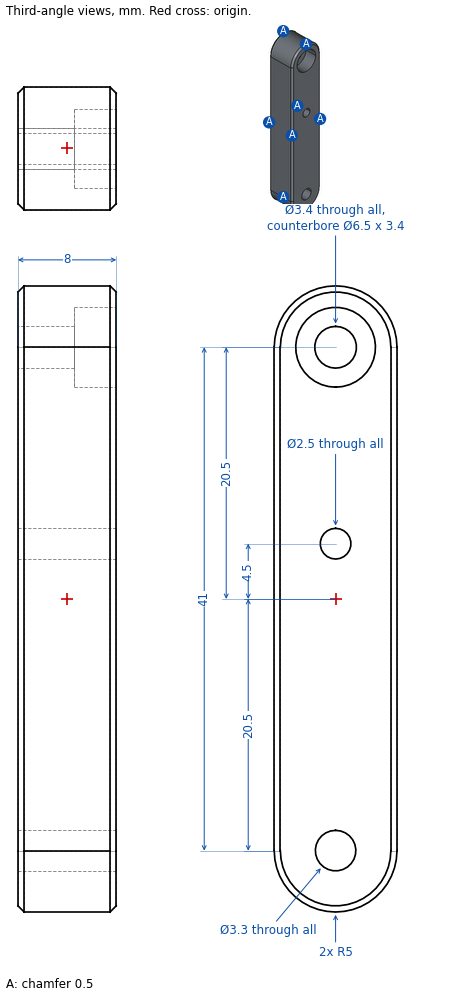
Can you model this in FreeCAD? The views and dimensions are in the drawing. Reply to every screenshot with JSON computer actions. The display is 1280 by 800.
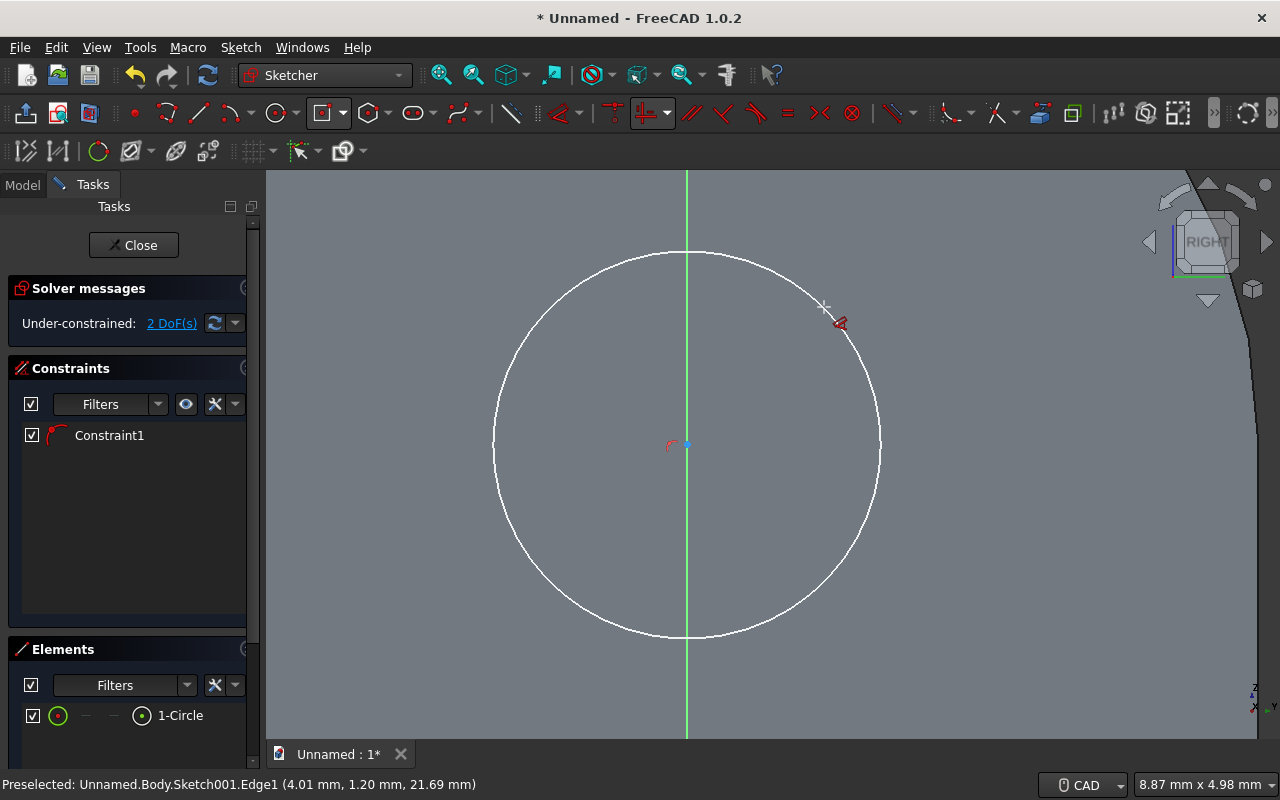
{"action": "left_click", "coordinate": [824, 308]}
{"action": "left_click", "coordinate": [847, 285]}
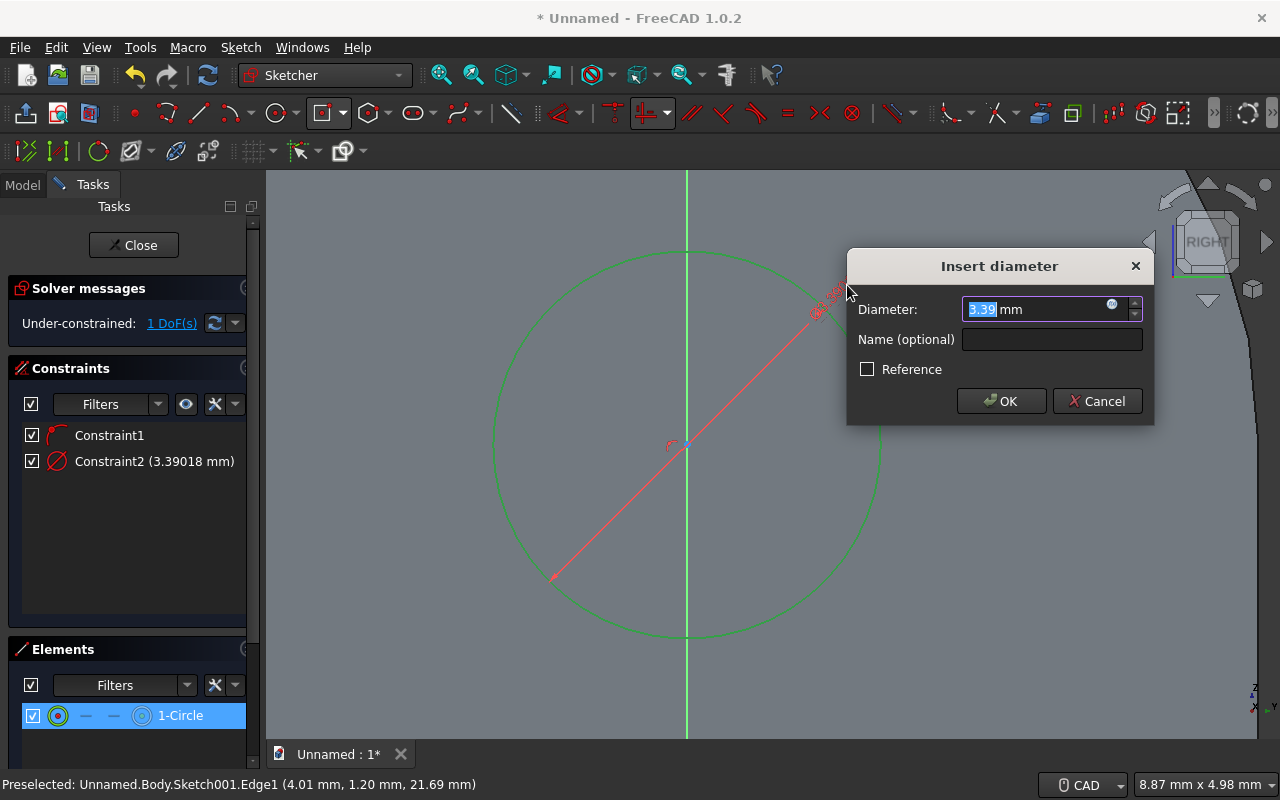
{"action": "type", "text": "3.4"}
{"action": "key", "text": "Return"}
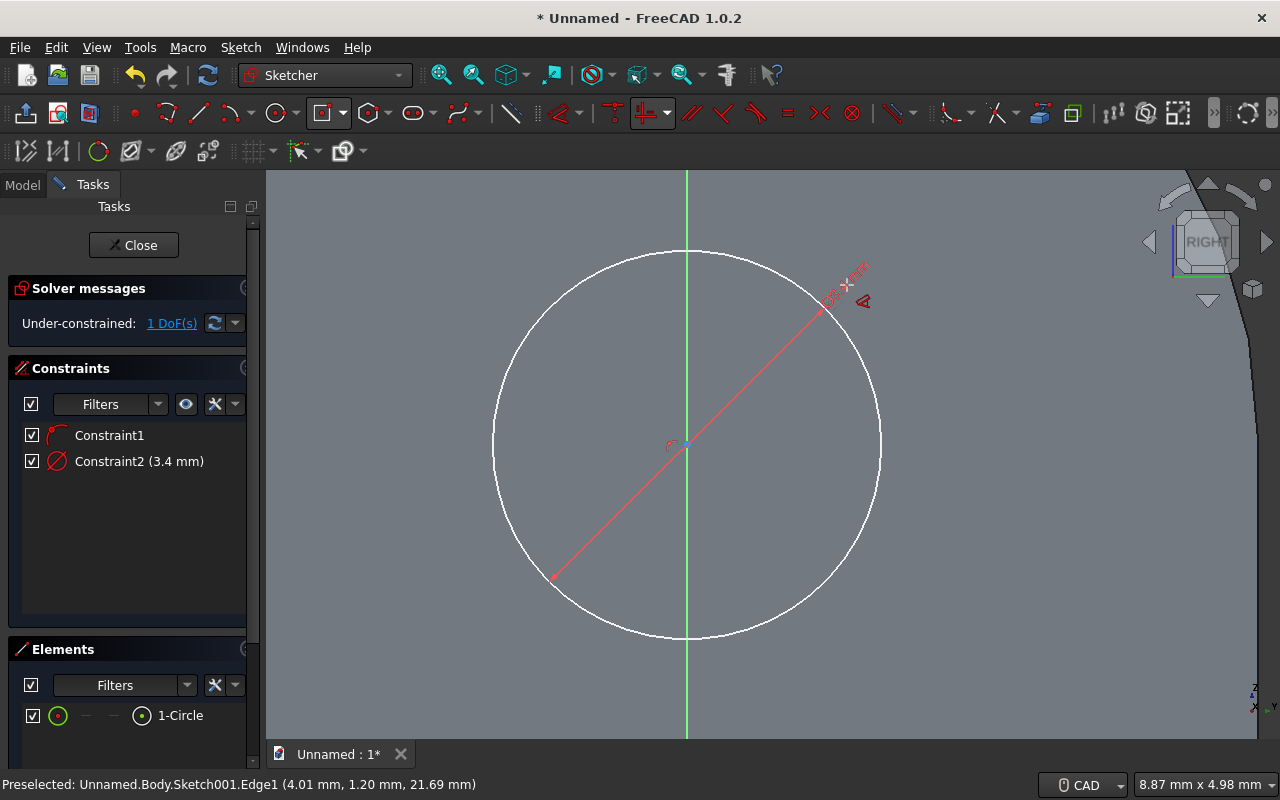
{"action": "left_click", "coordinate": [687, 445]}
{"action": "left_click", "coordinate": [721, 578]}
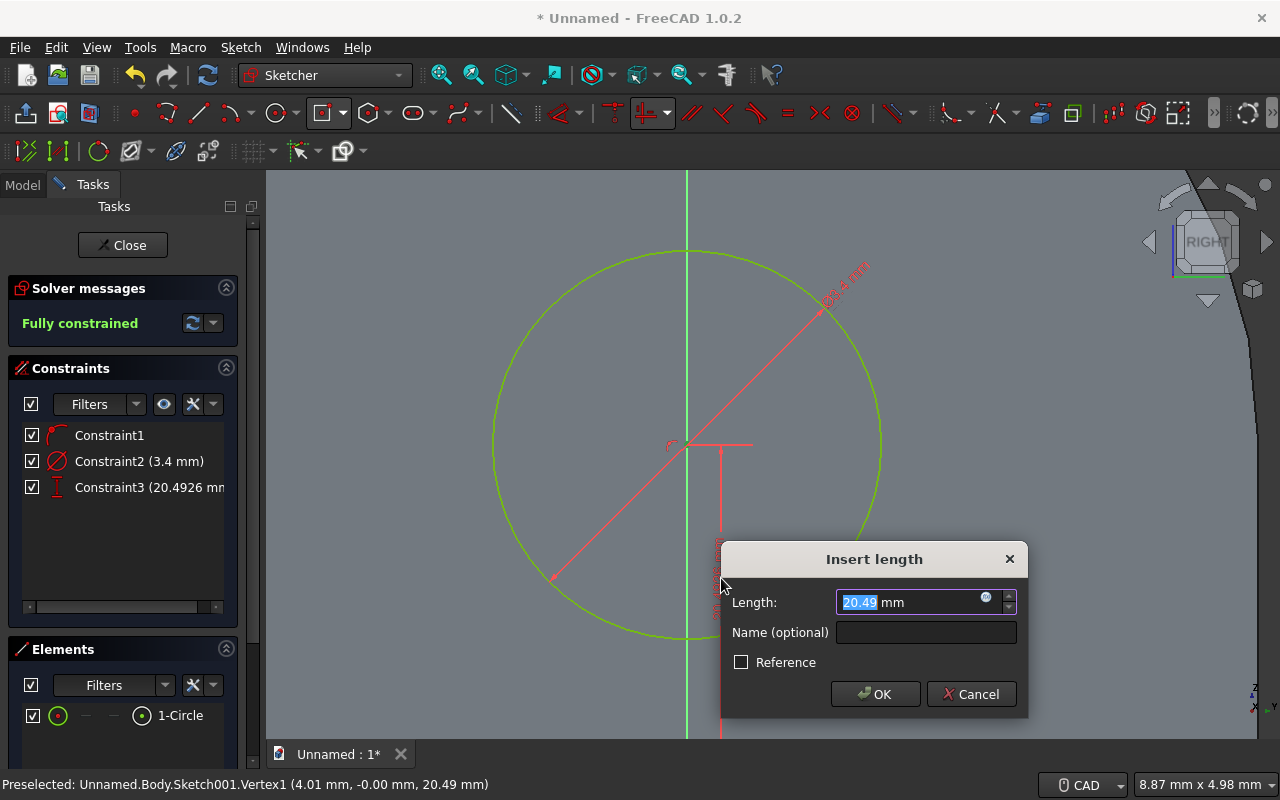
{"action": "type", "text": "20.5"}
{"action": "key", "text": "Return"}
{"action": "key", "text": "Escape"}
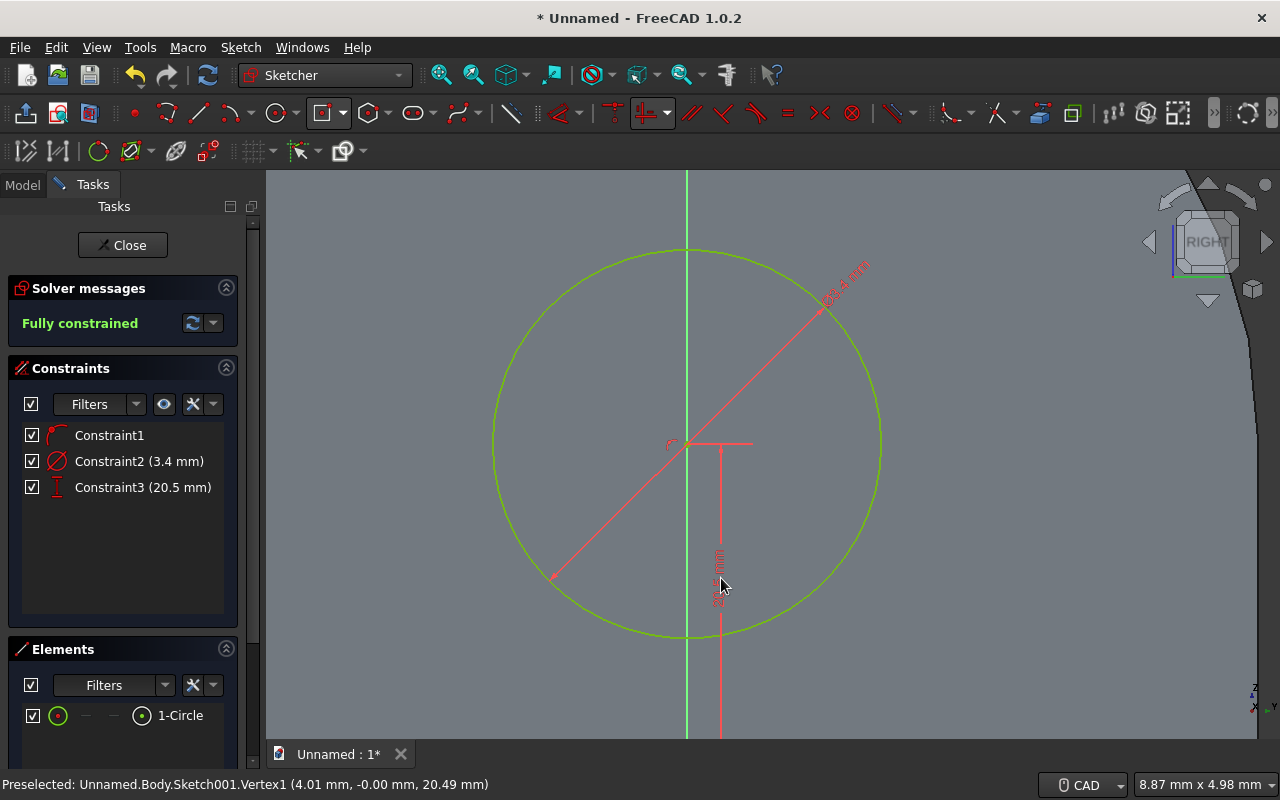
{"action": "left_click", "coordinate": [123, 245]}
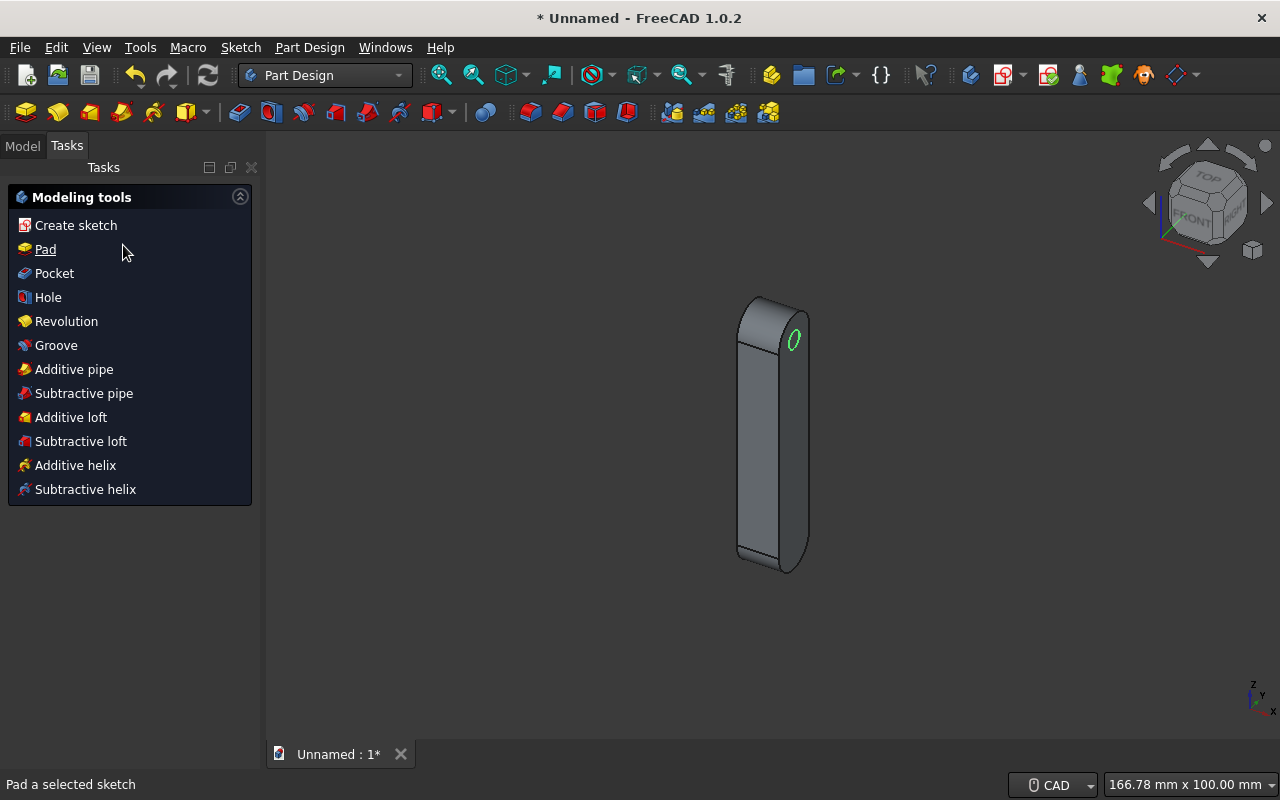
{"action": "left_click", "coordinate": [272, 112]}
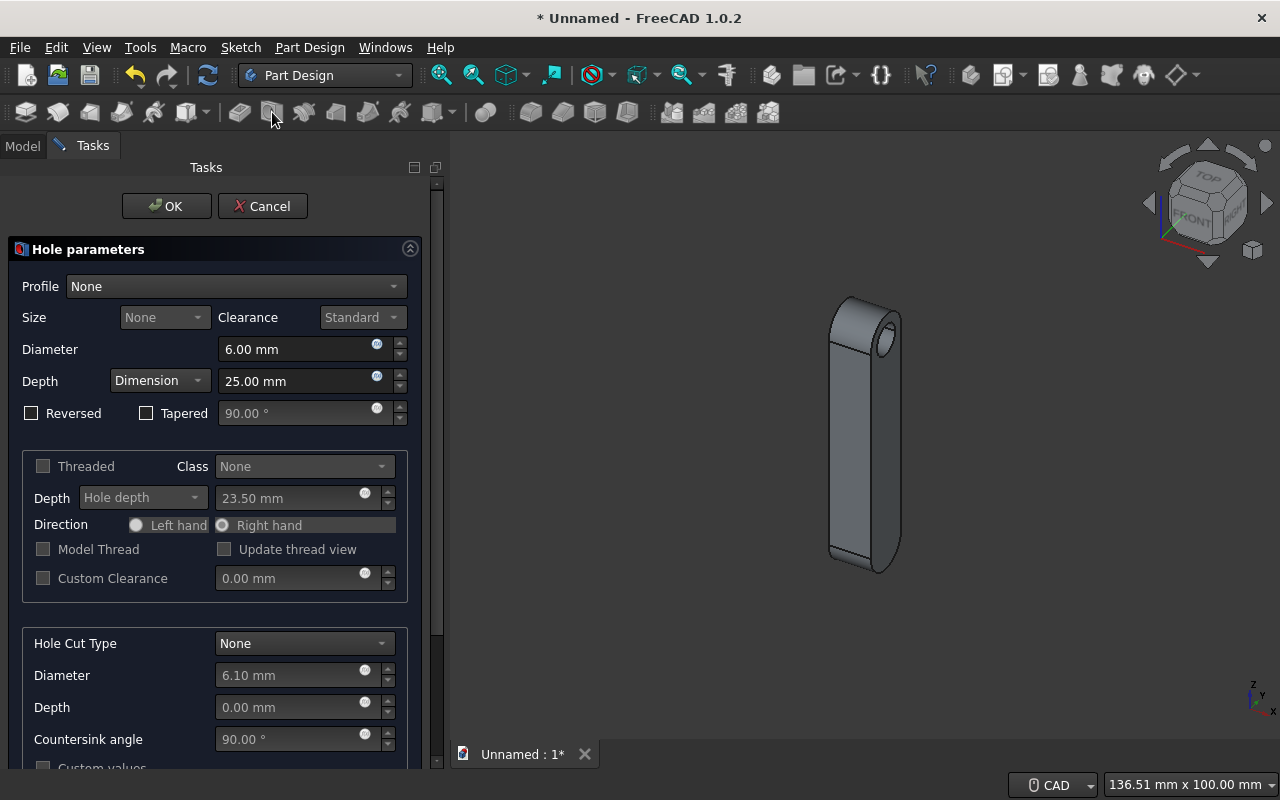
{"action": "triple_click", "coordinate": [305, 349]}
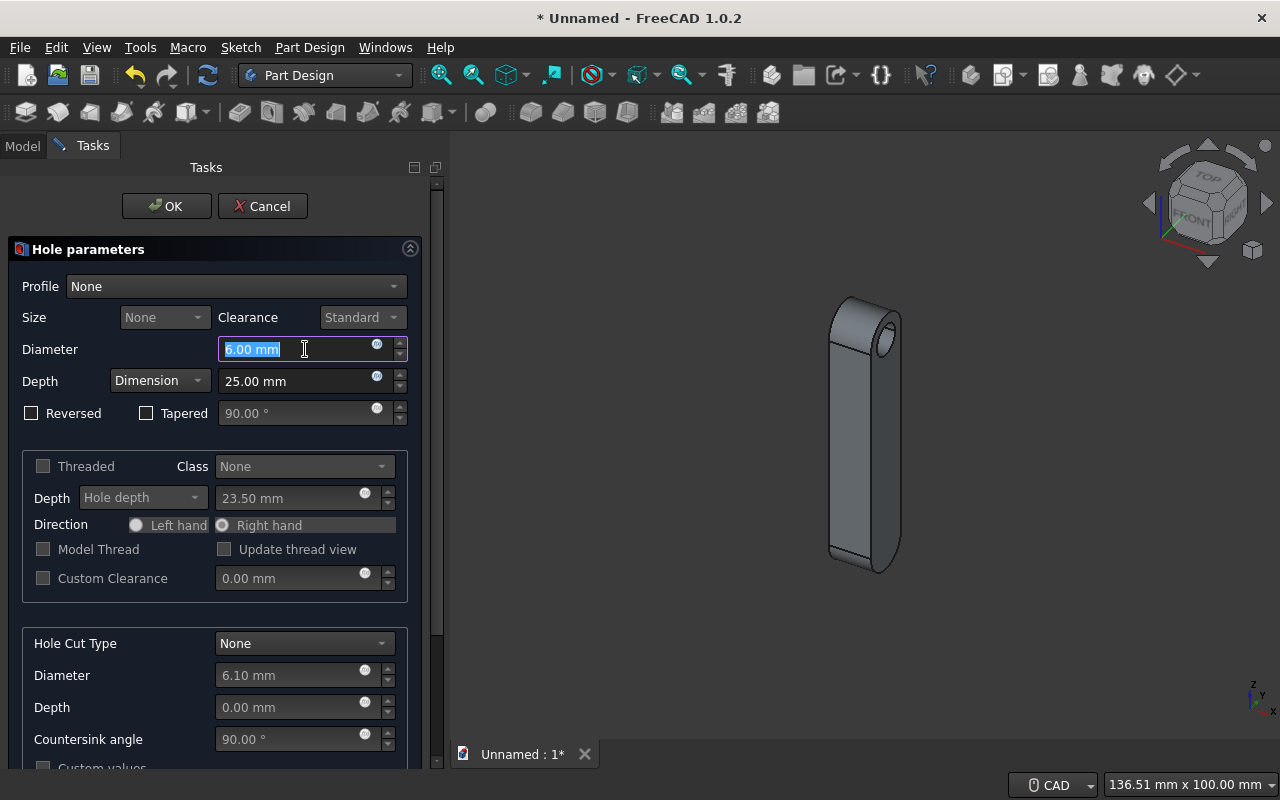
{"action": "type", "text": "3.4"}
{"action": "key", "text": "Tab"}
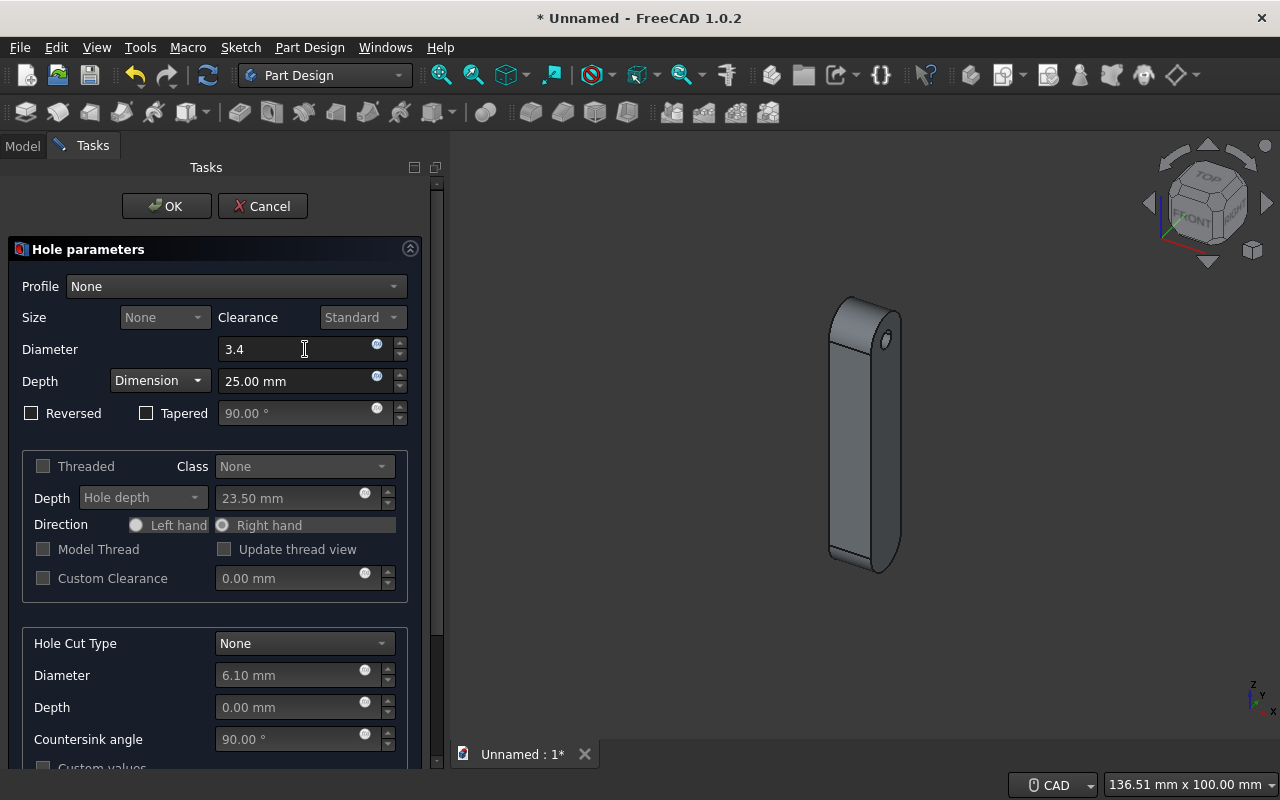
{"action": "left_click", "coordinate": [161, 380]}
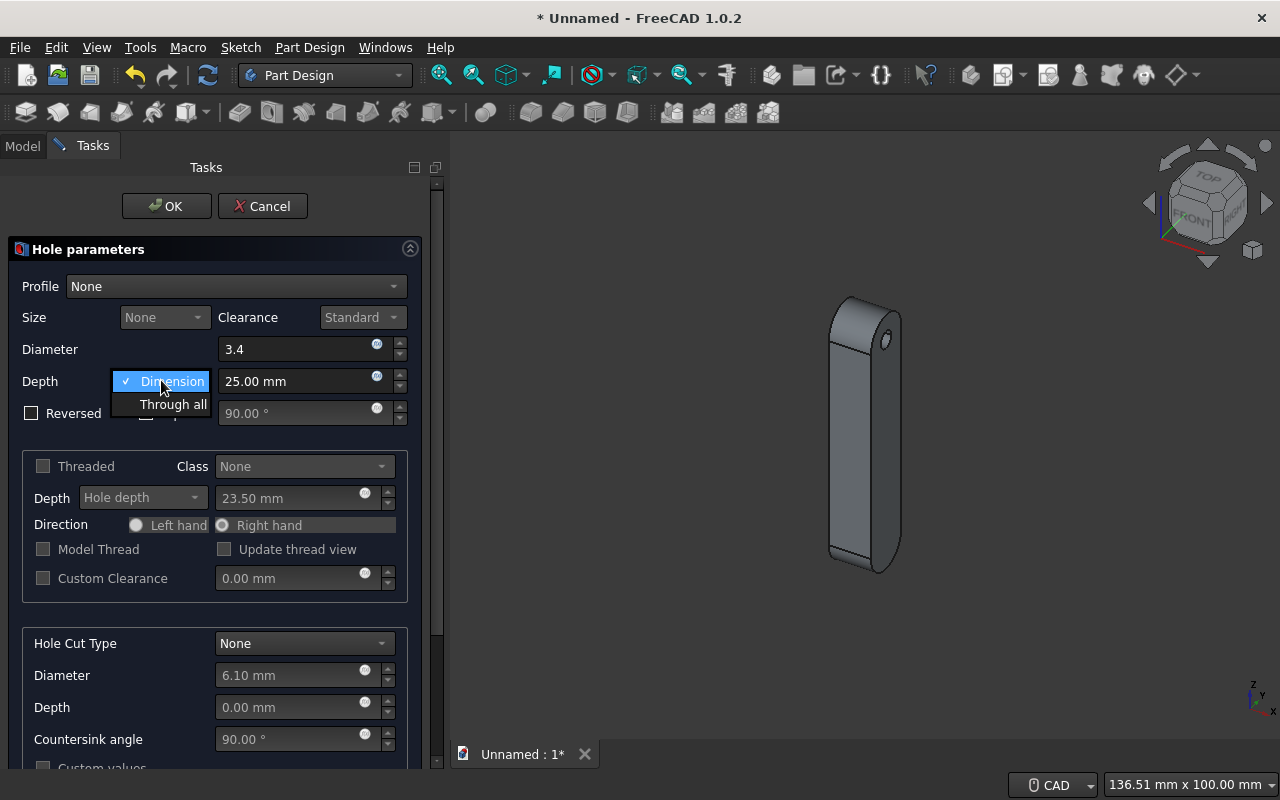
{"action": "left_click", "coordinate": [160, 404]}